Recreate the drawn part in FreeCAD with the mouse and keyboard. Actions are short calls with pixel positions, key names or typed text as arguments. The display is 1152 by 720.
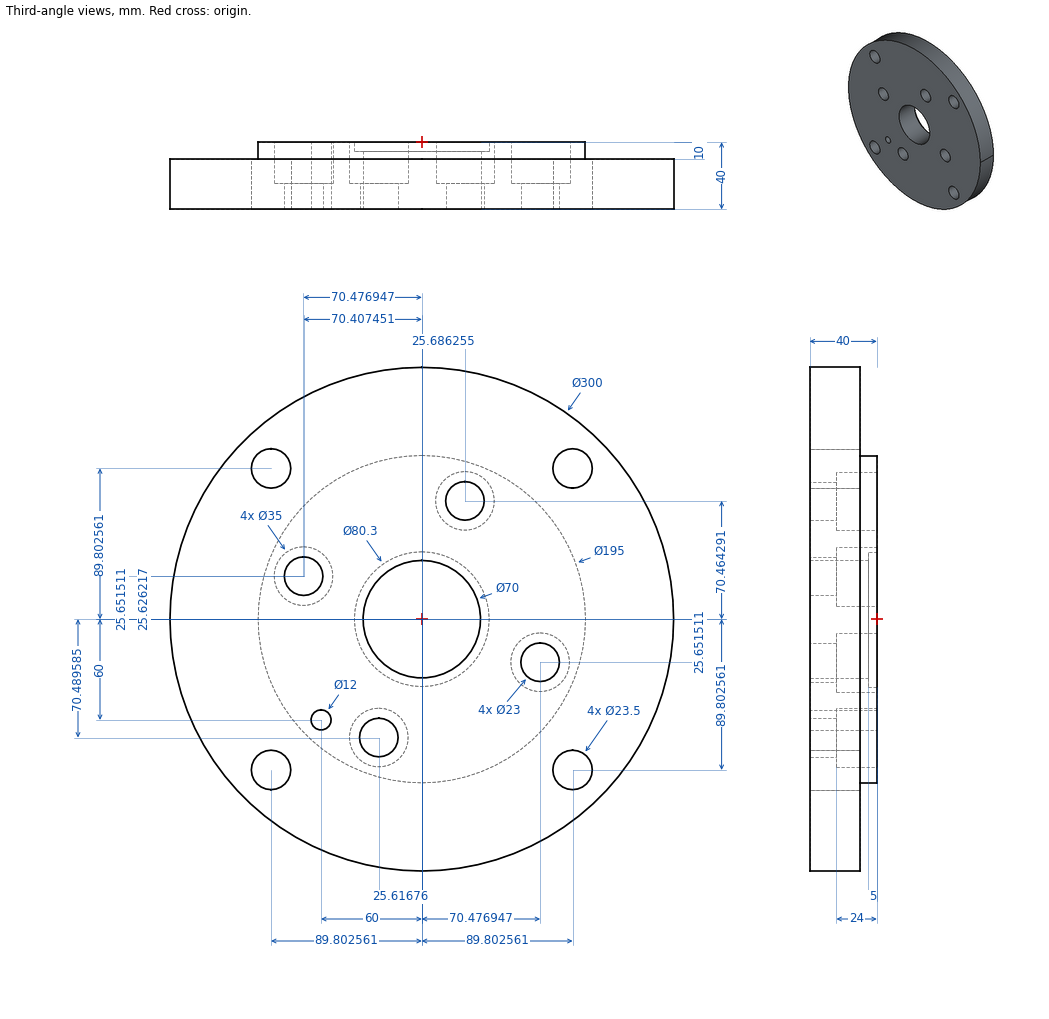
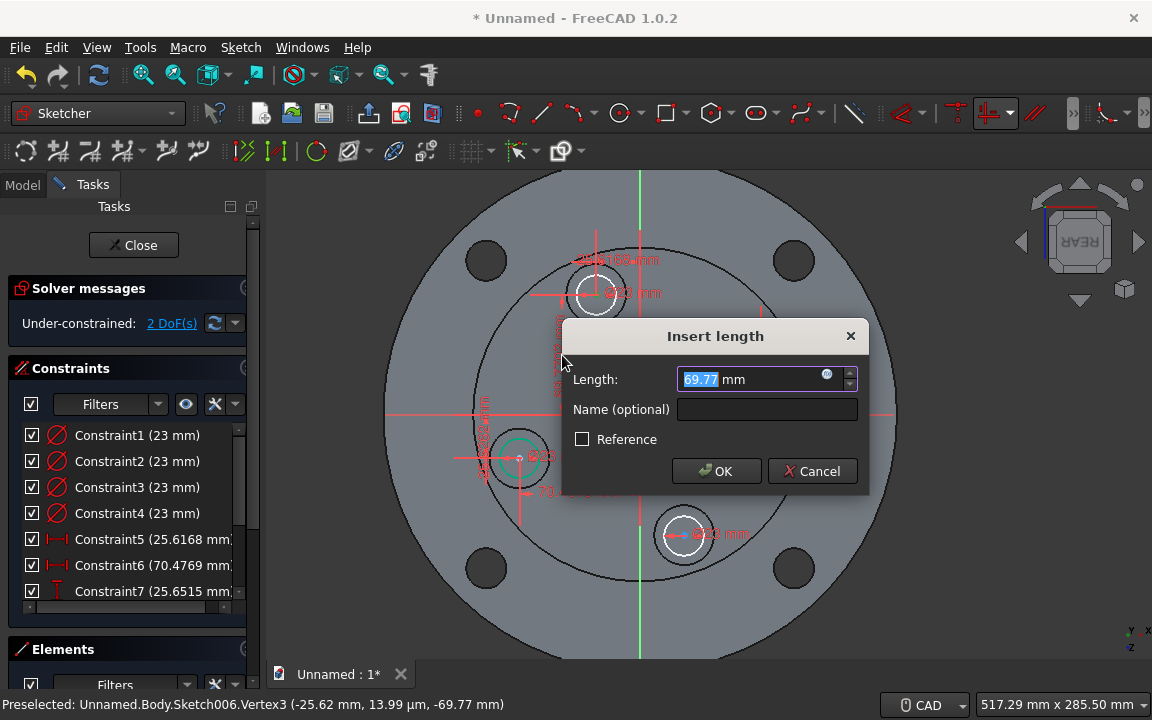
text(70.489585)
key(Return)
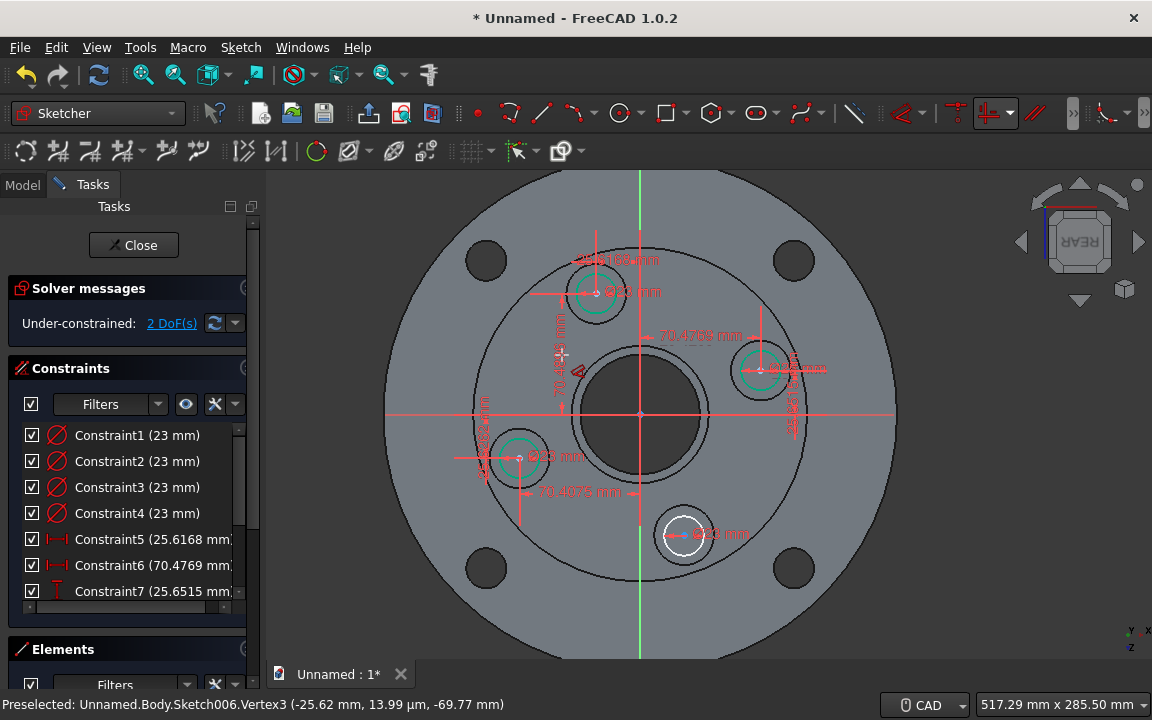
click(684, 536)
click(662, 570)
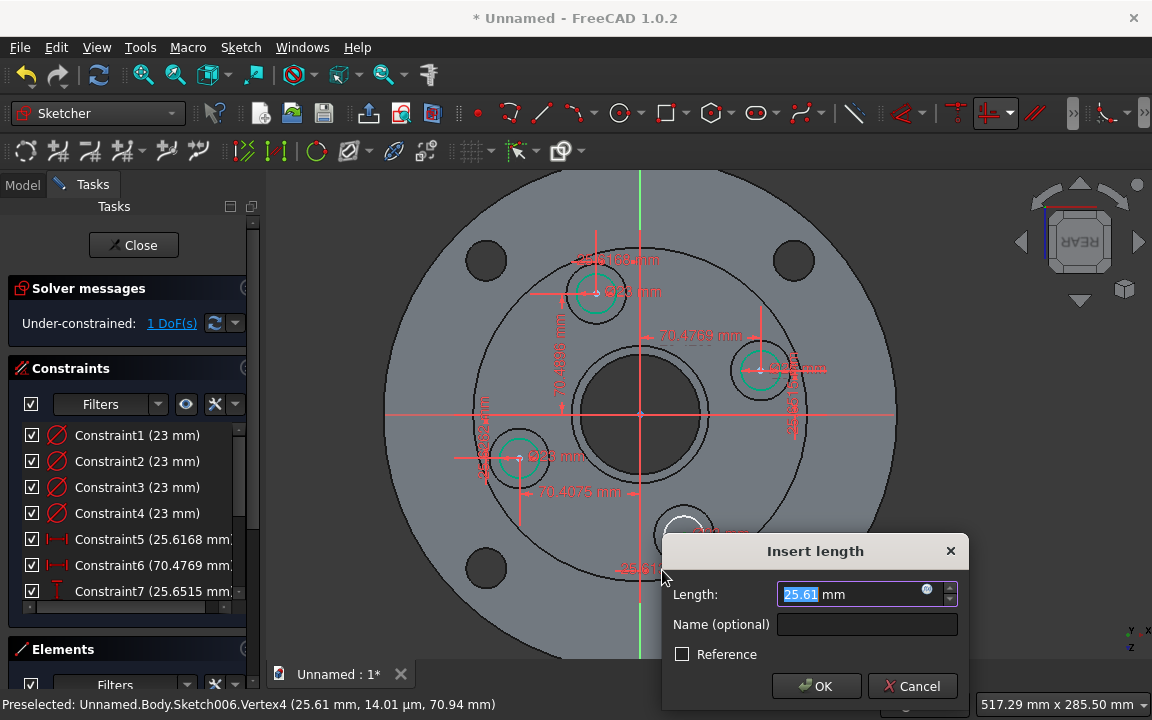
text(25.686255)
key(Return)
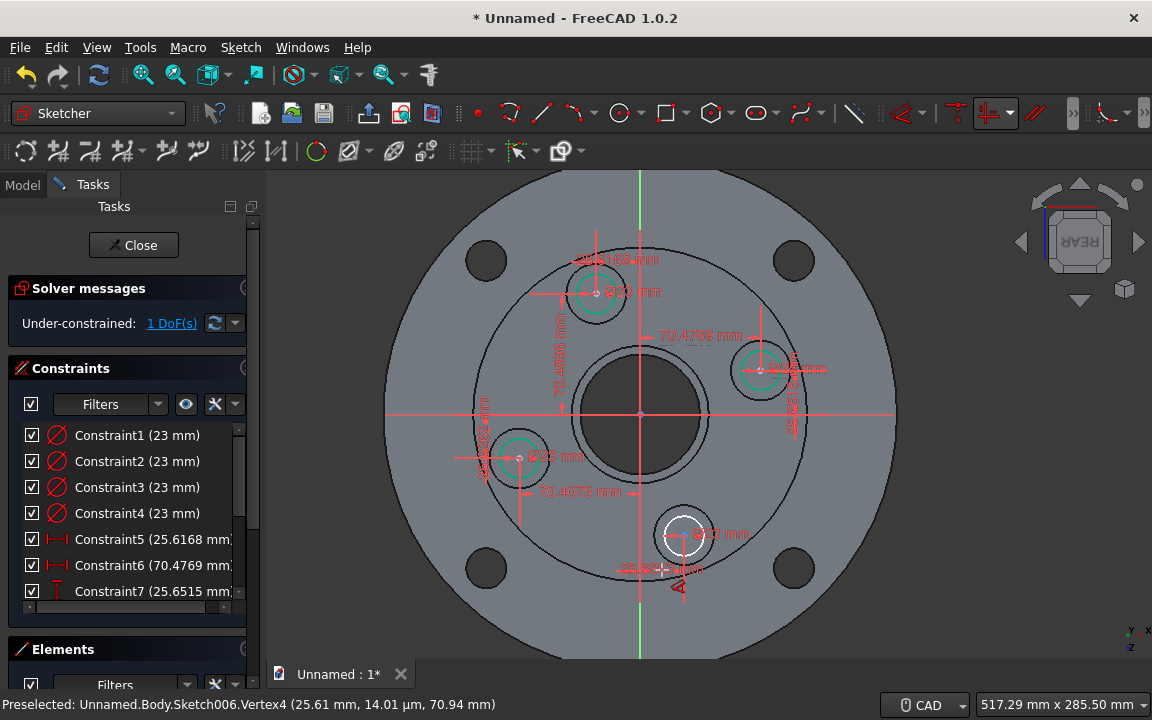
click(684, 536)
click(718, 475)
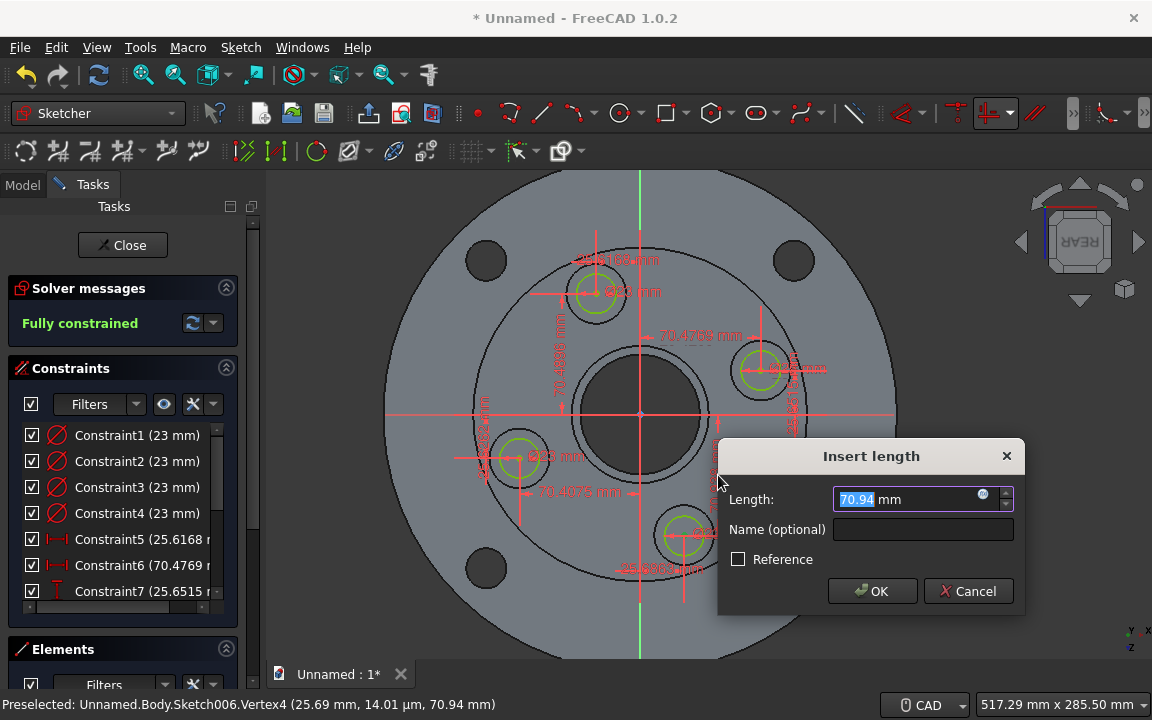
text(70.464291)
key(Return)
key(Escape)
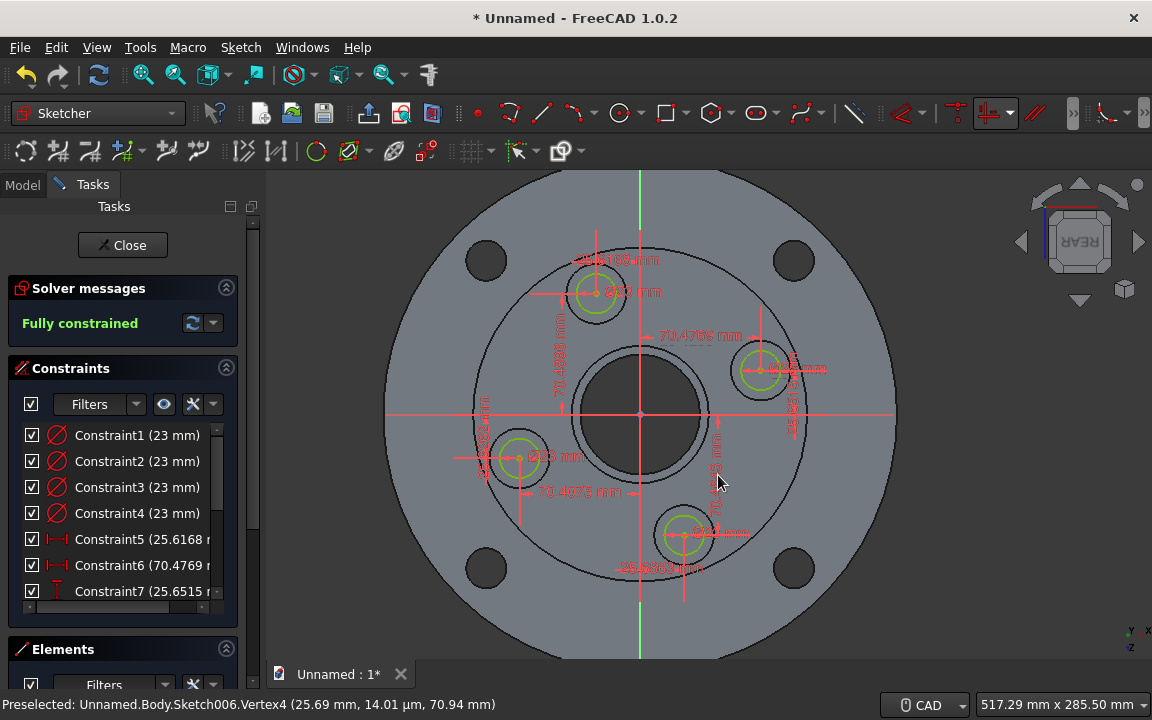
click(123, 245)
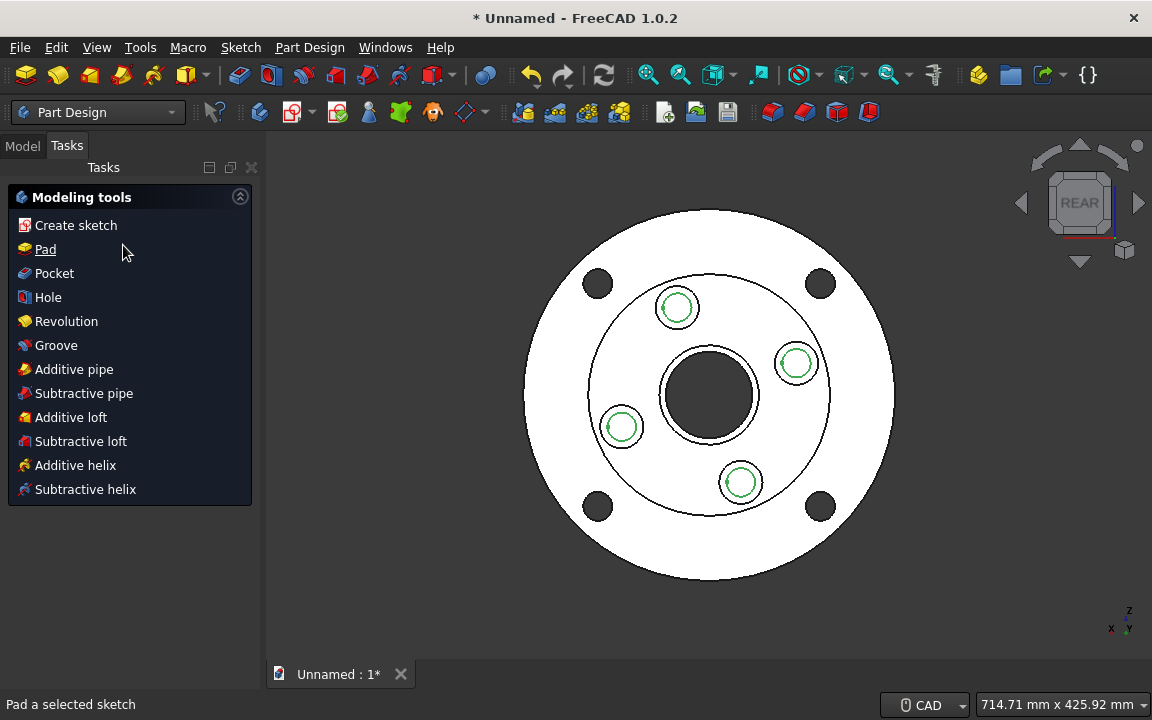
click(240, 76)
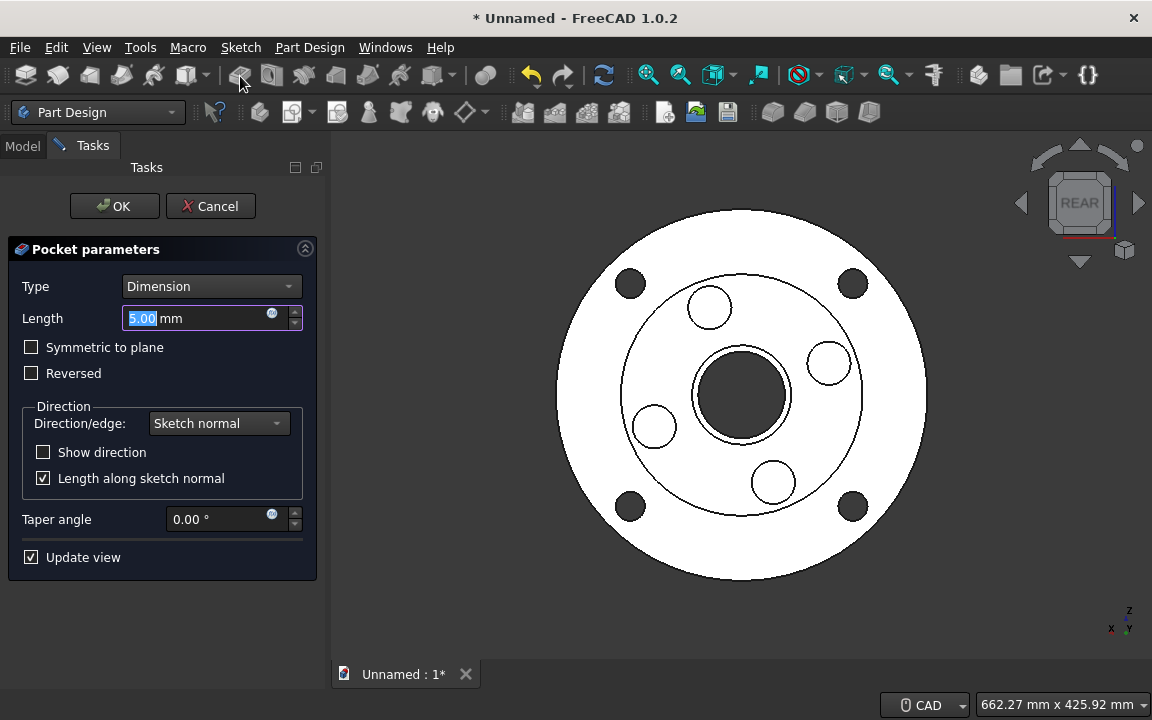
click(212, 286)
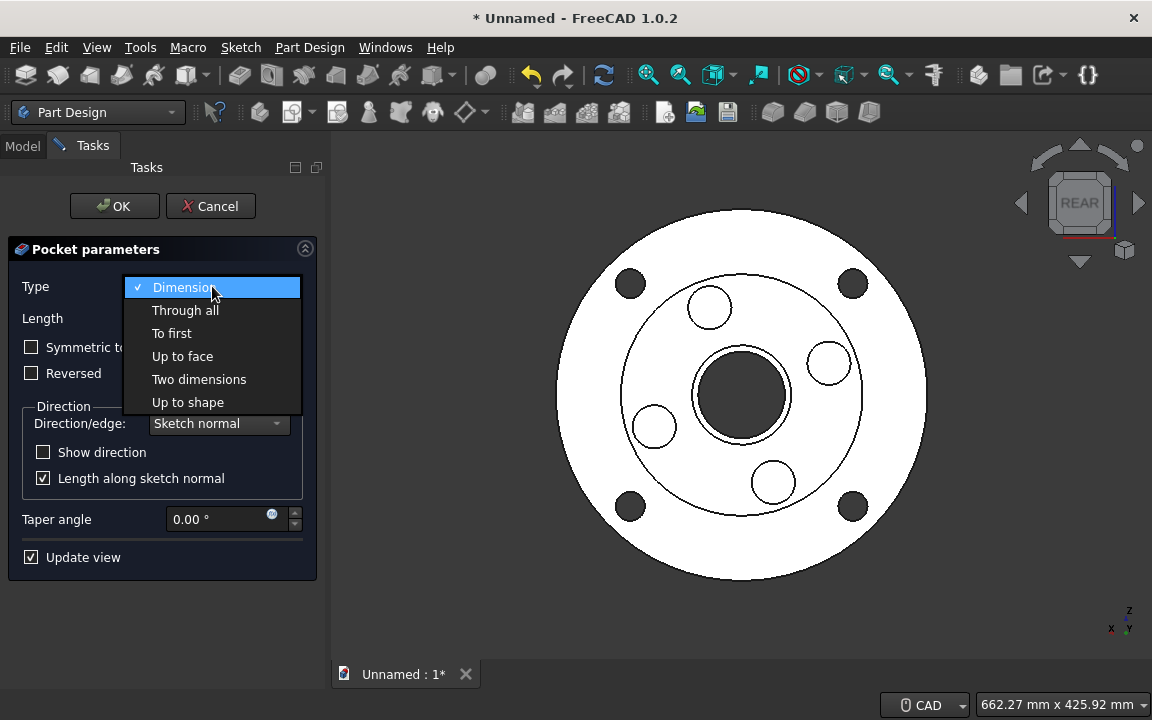
click(212, 310)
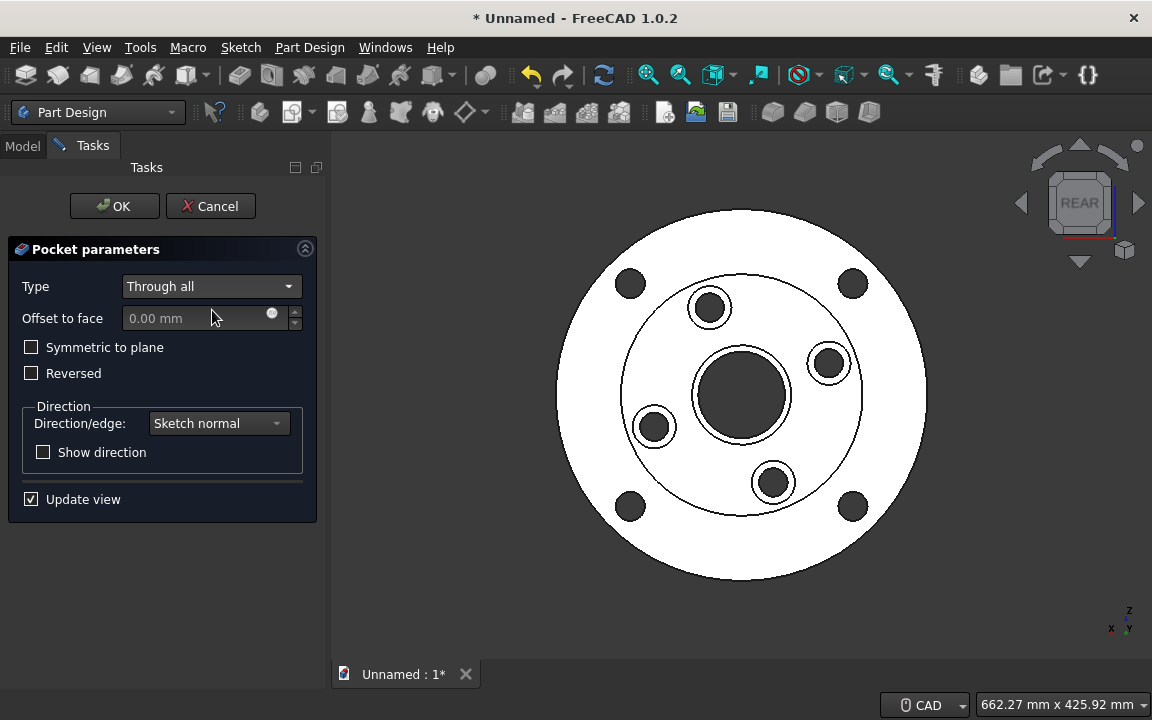
click(115, 206)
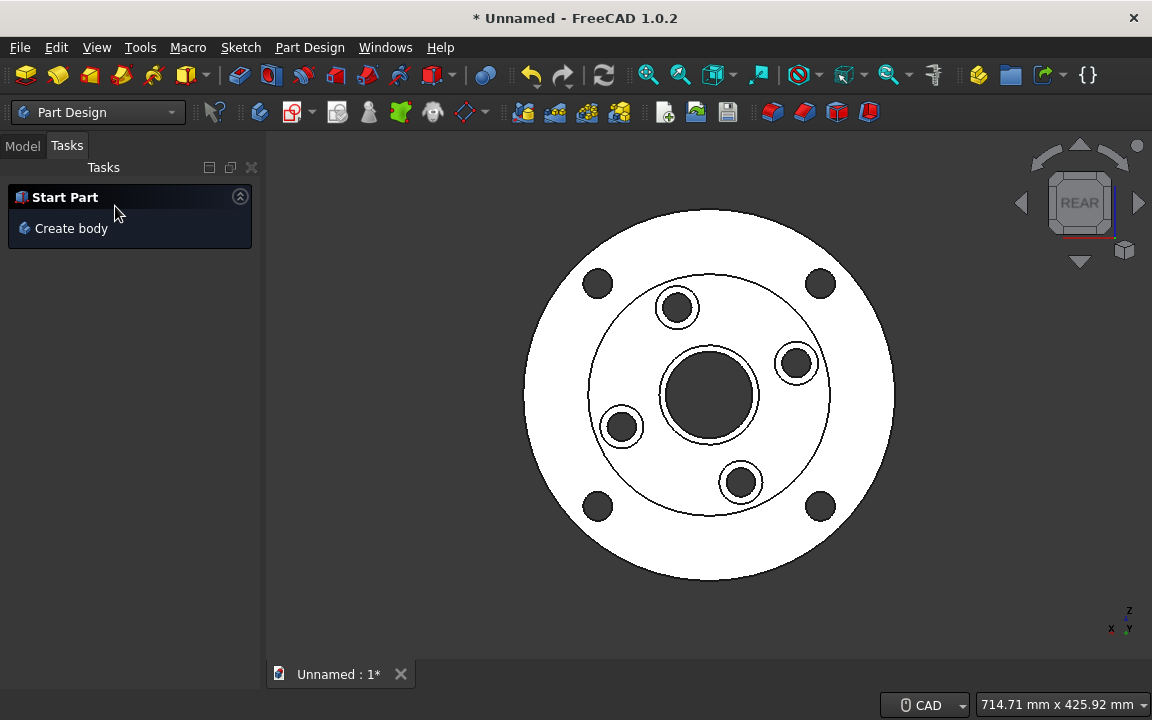
click(640, 359)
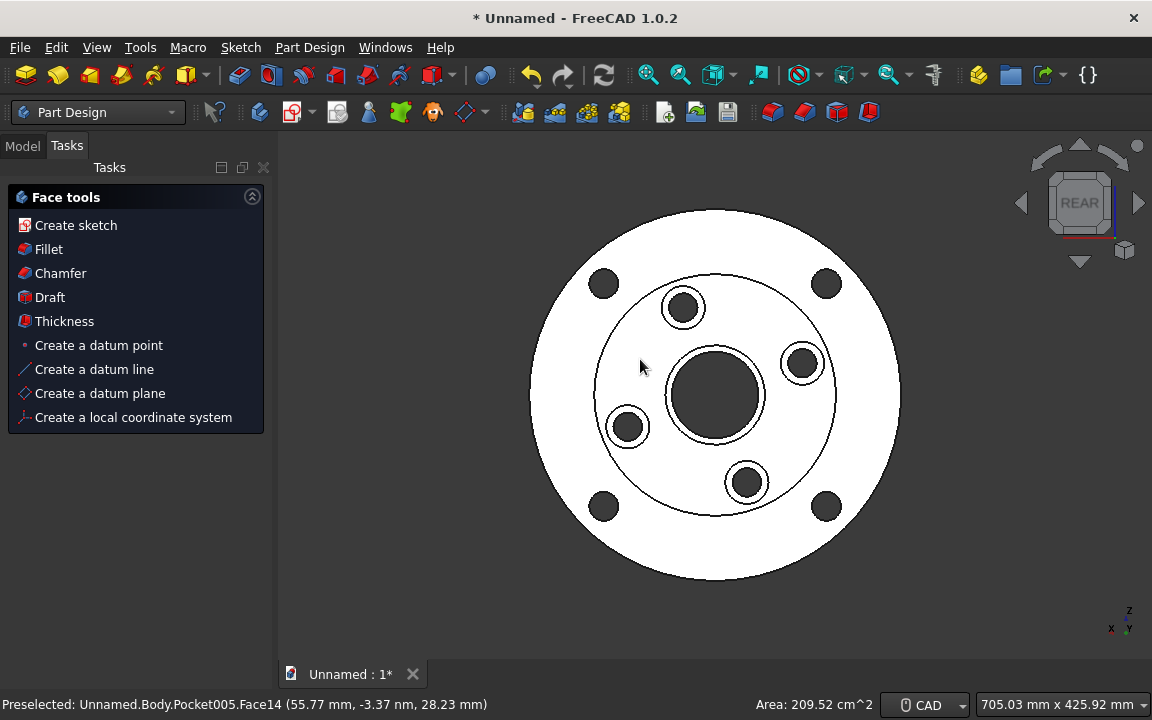
click(292, 112)